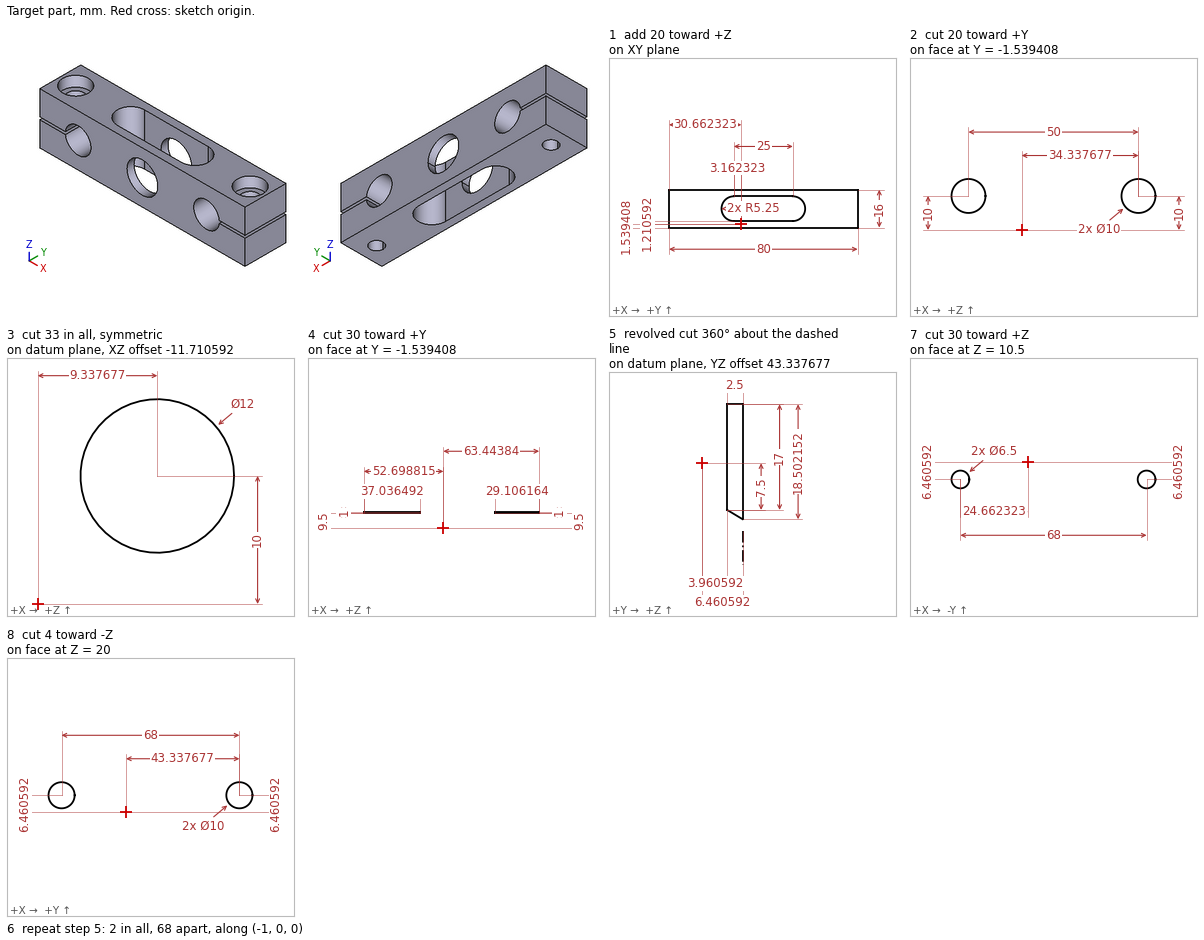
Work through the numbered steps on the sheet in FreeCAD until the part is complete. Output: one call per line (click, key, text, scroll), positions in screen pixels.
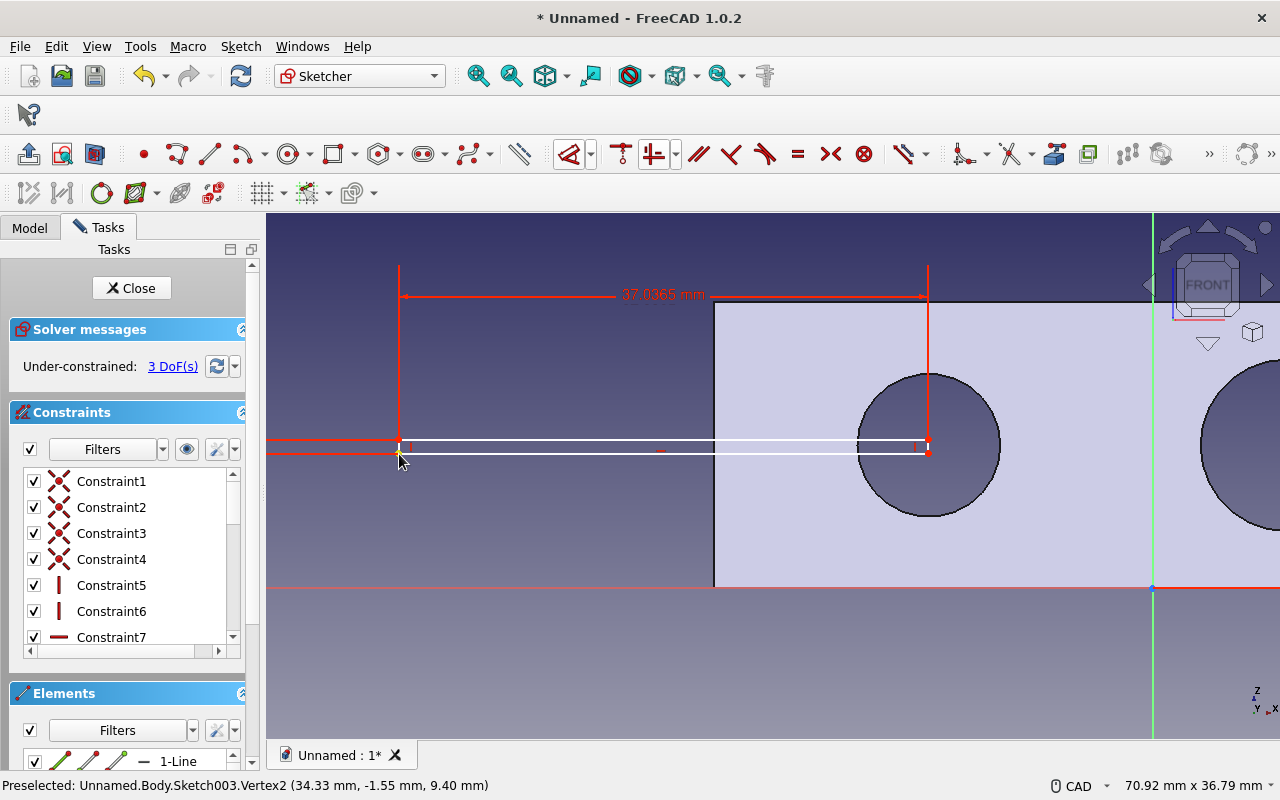
click(399, 454)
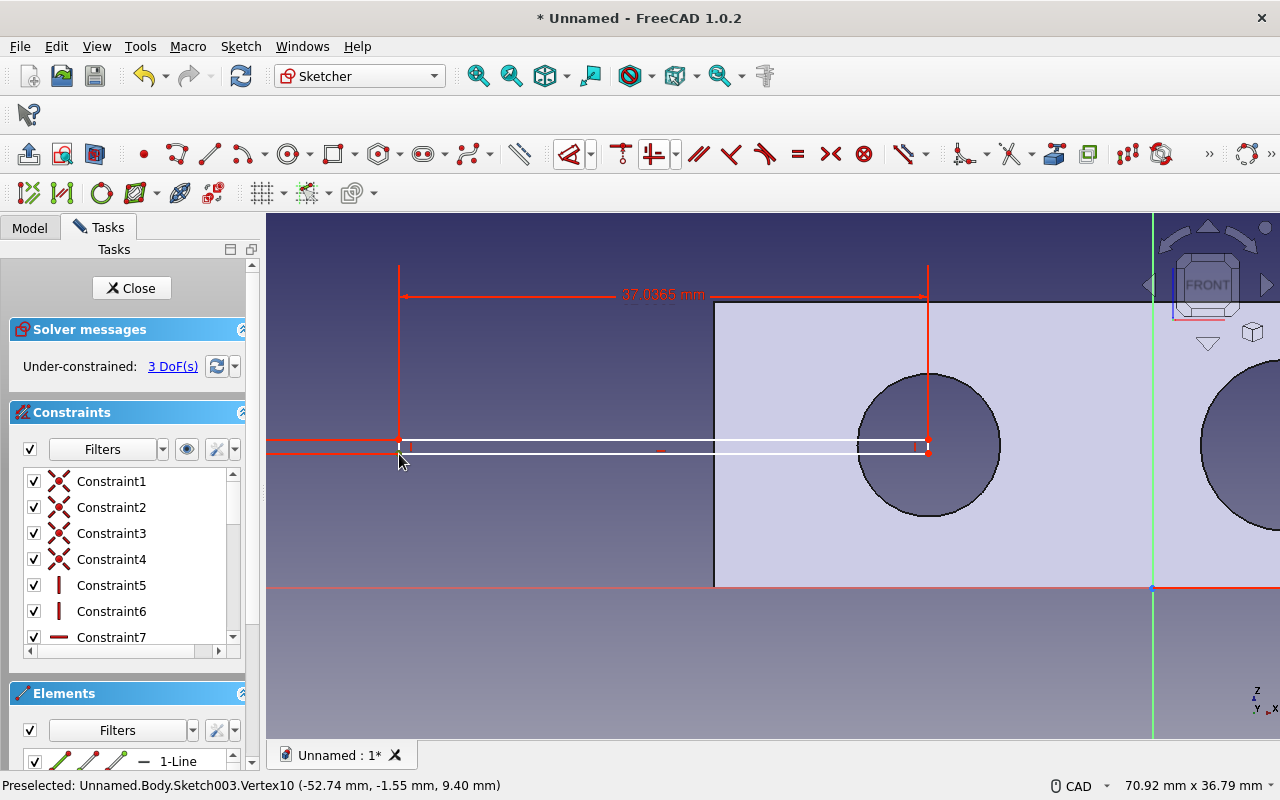
click(590, 154)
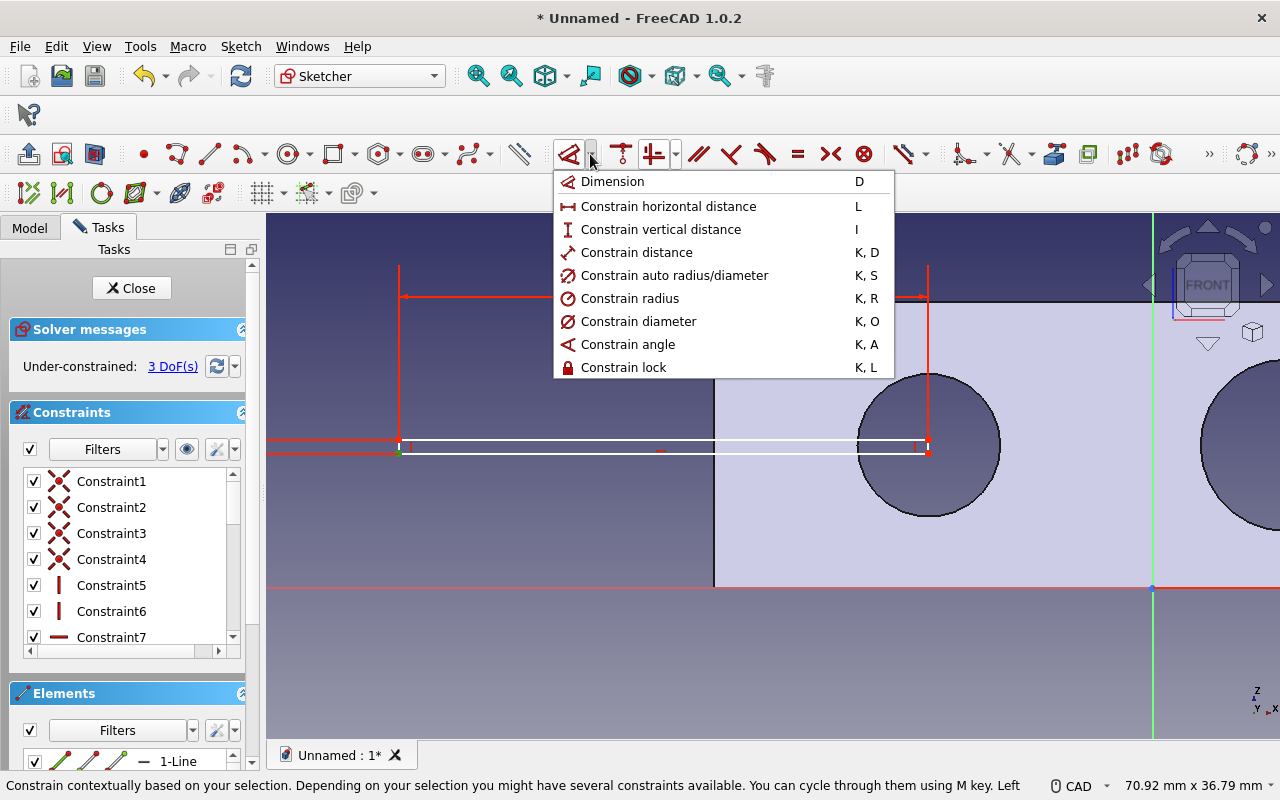
click(724, 230)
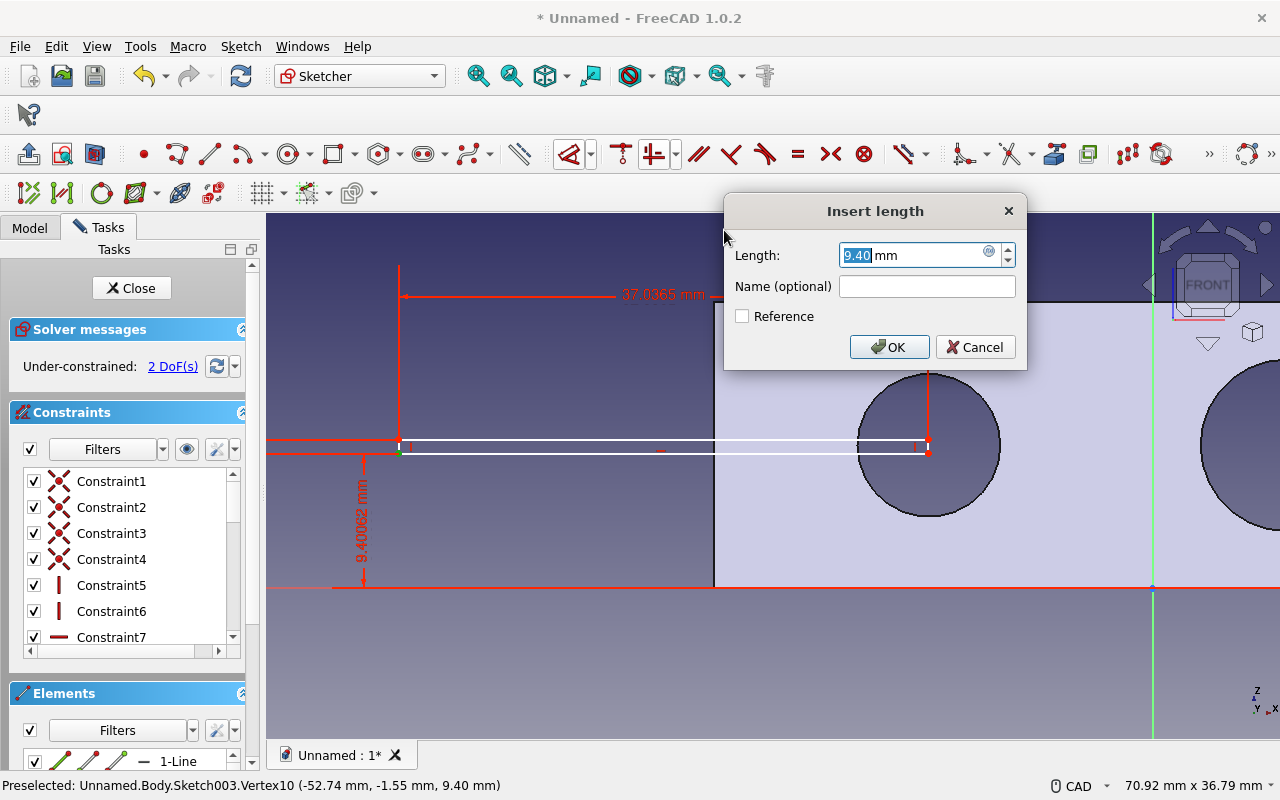
text(9.5)
key(Return)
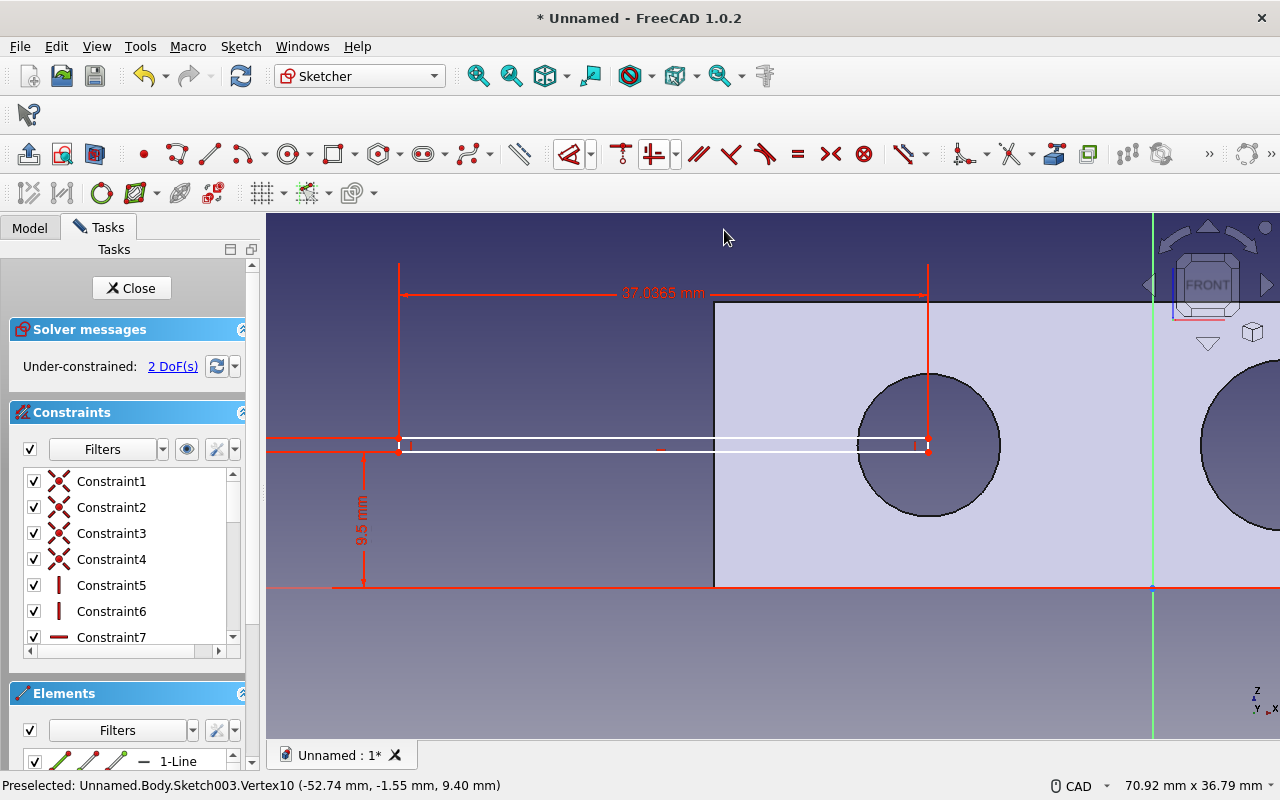
scroll(399, 454, down, 5)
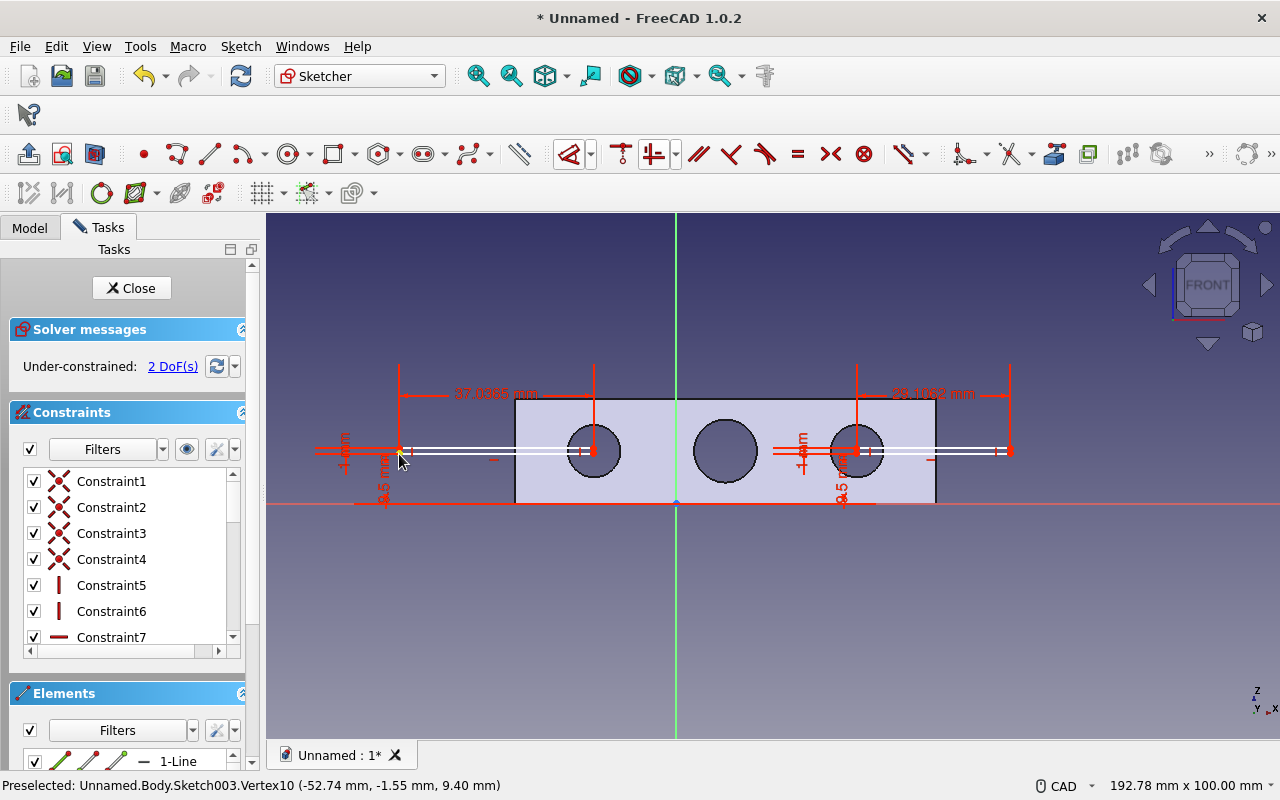
scroll(1010, 454, up, 5)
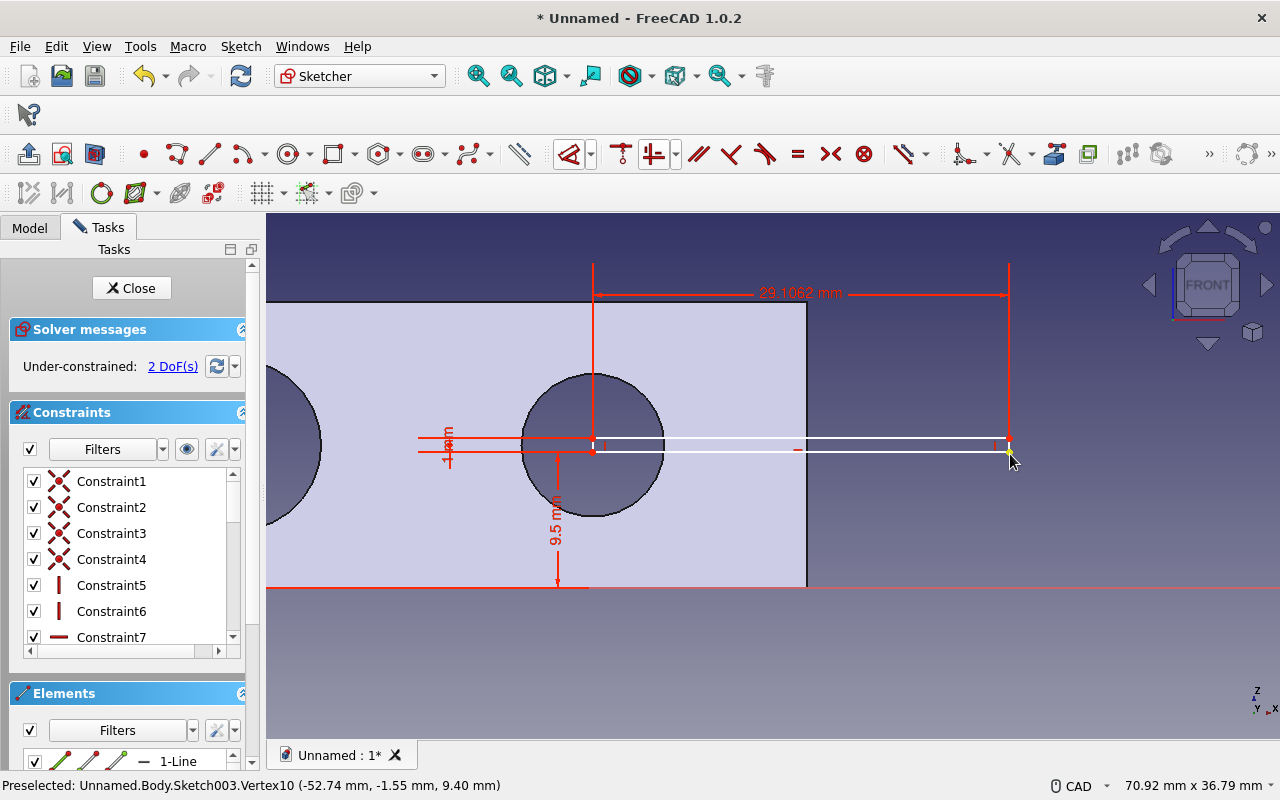
click(1009, 452)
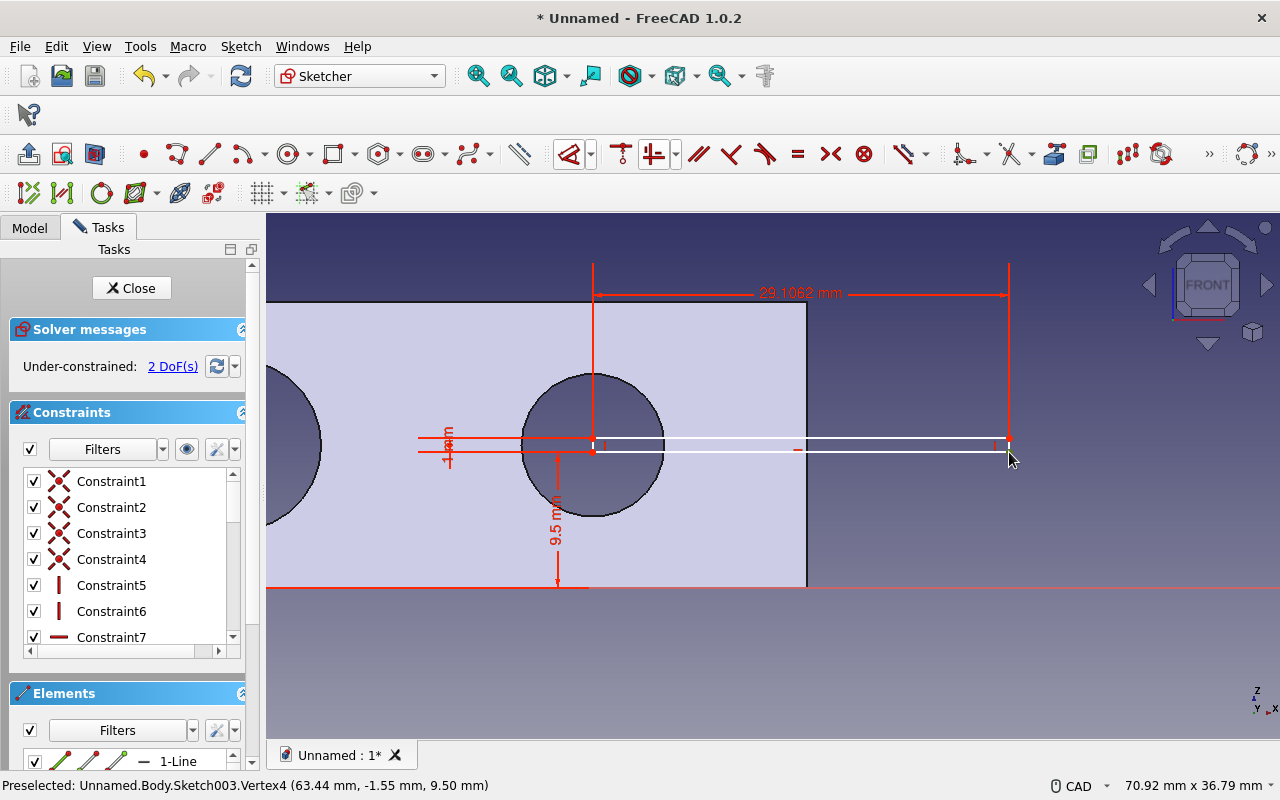
key(l)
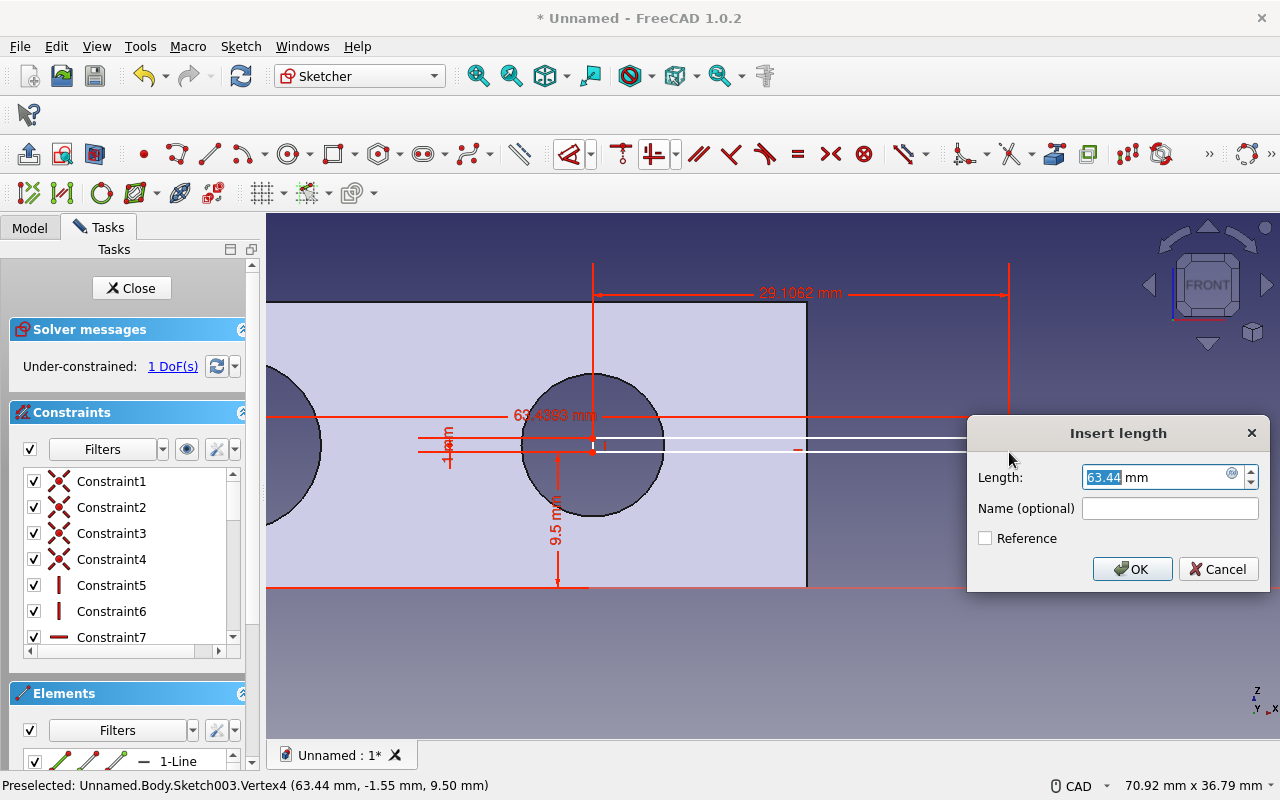
text(63.44384)
key(Return)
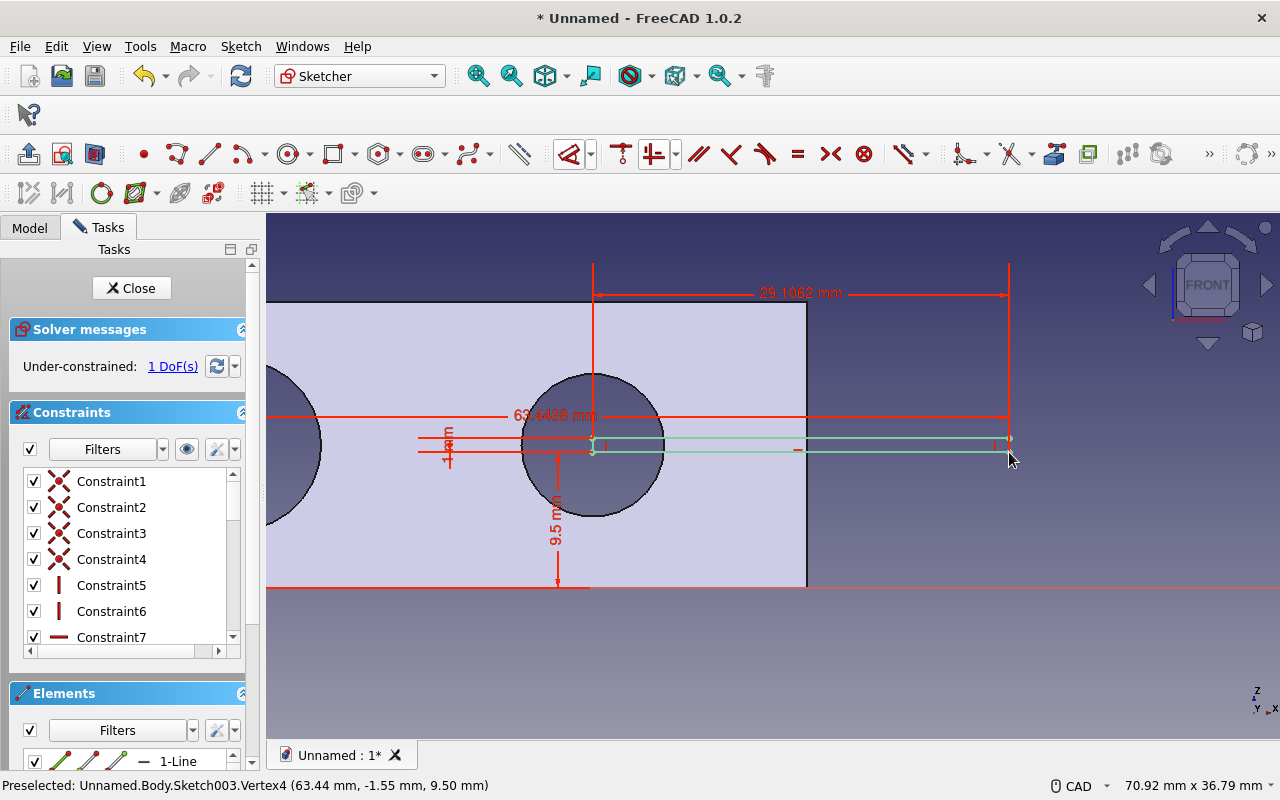
scroll(1010, 454, down, 5)